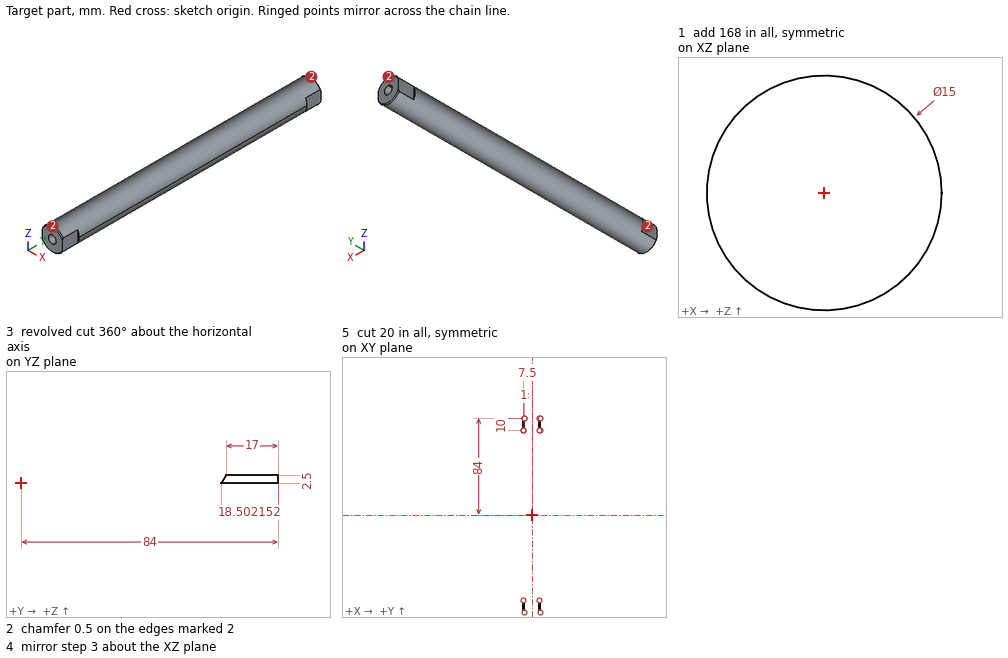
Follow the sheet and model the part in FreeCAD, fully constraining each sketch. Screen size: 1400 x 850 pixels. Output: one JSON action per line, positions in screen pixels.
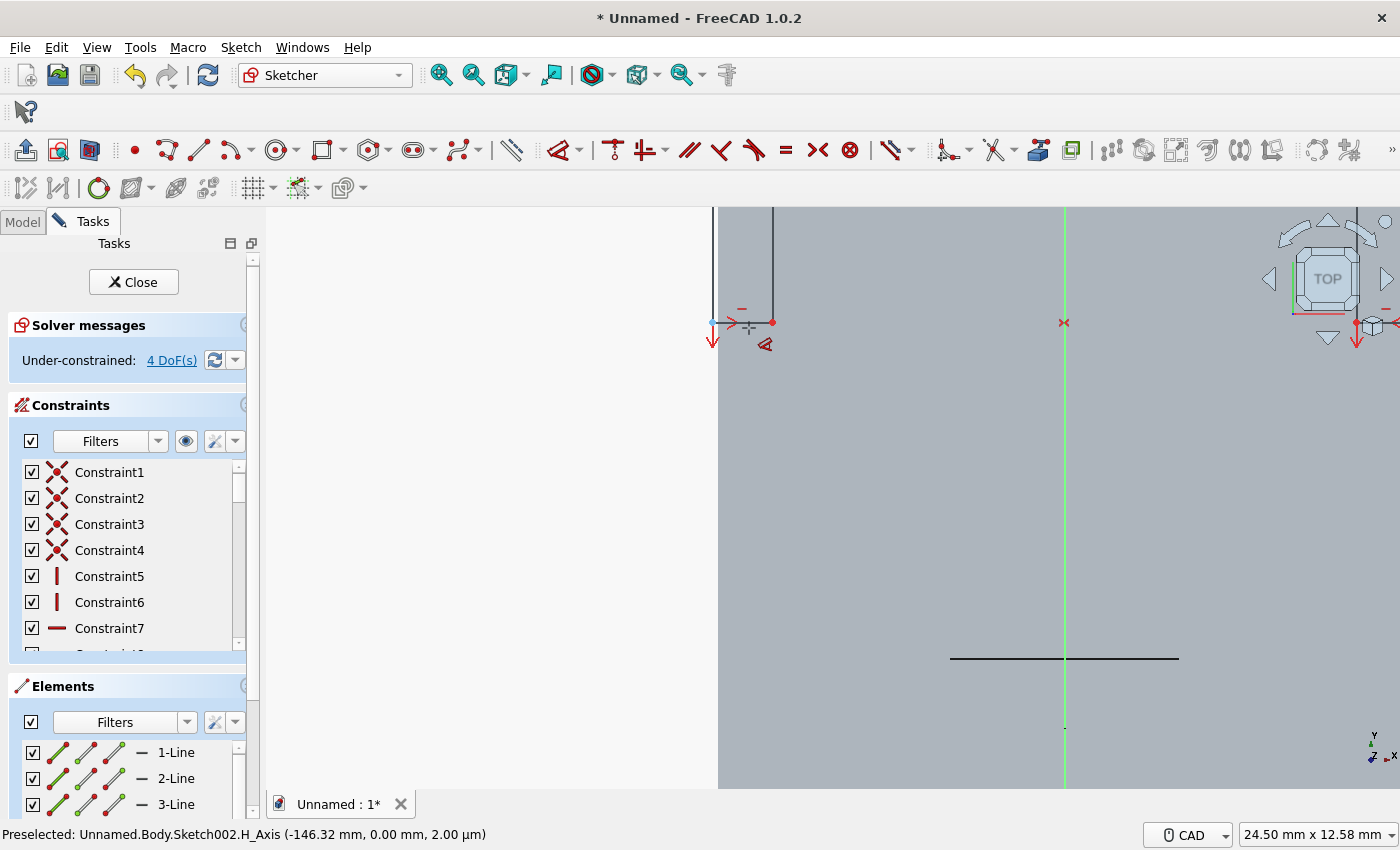
{"action": "left_click", "coordinate": [743, 323]}
{"action": "left_click", "coordinate": [743, 289]}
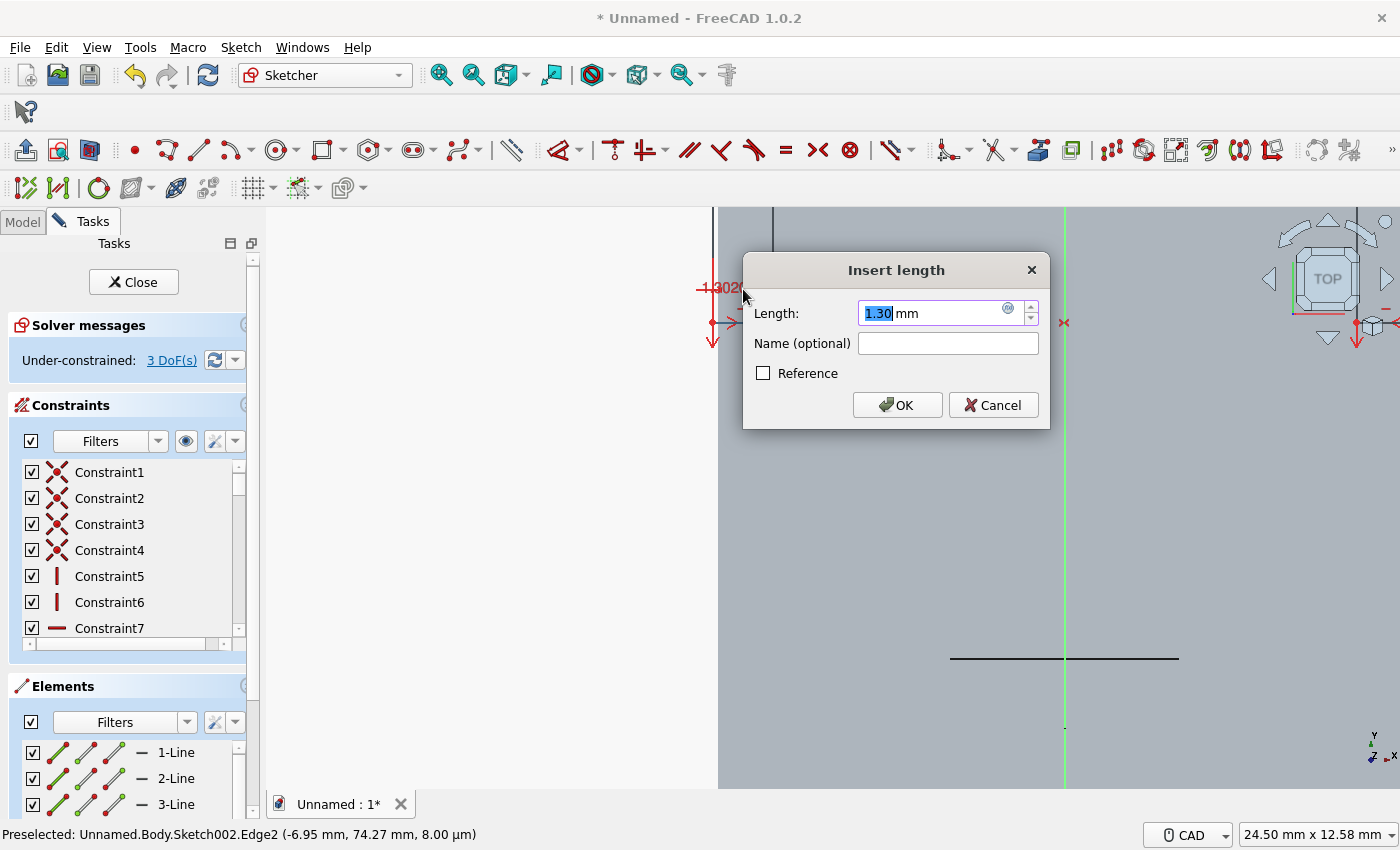
{"action": "type", "text": "1"}
{"action": "key", "text": "Return"}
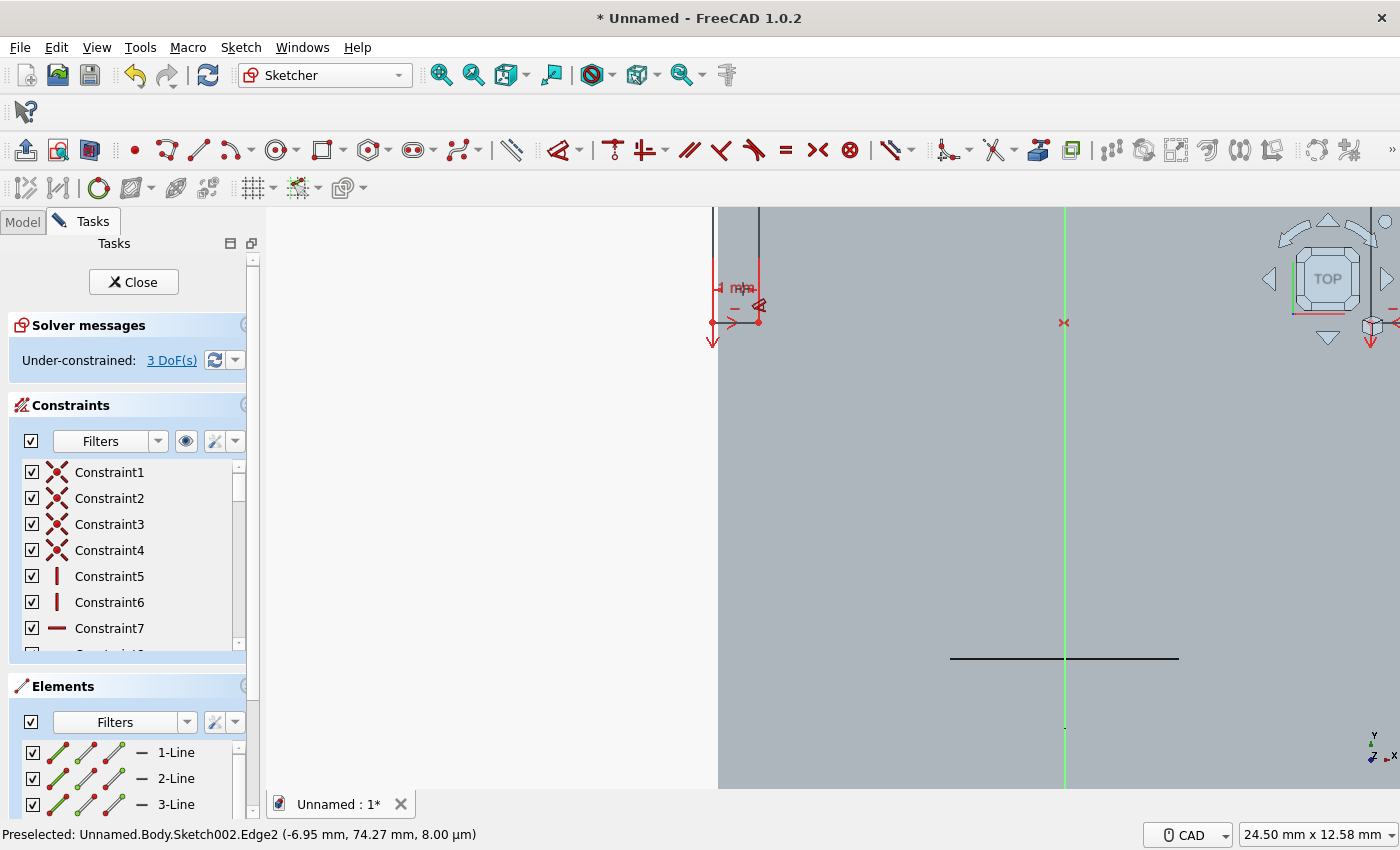
{"action": "scroll", "coordinate": [749, 327], "scroll_direction": "down", "scroll_amount": 15}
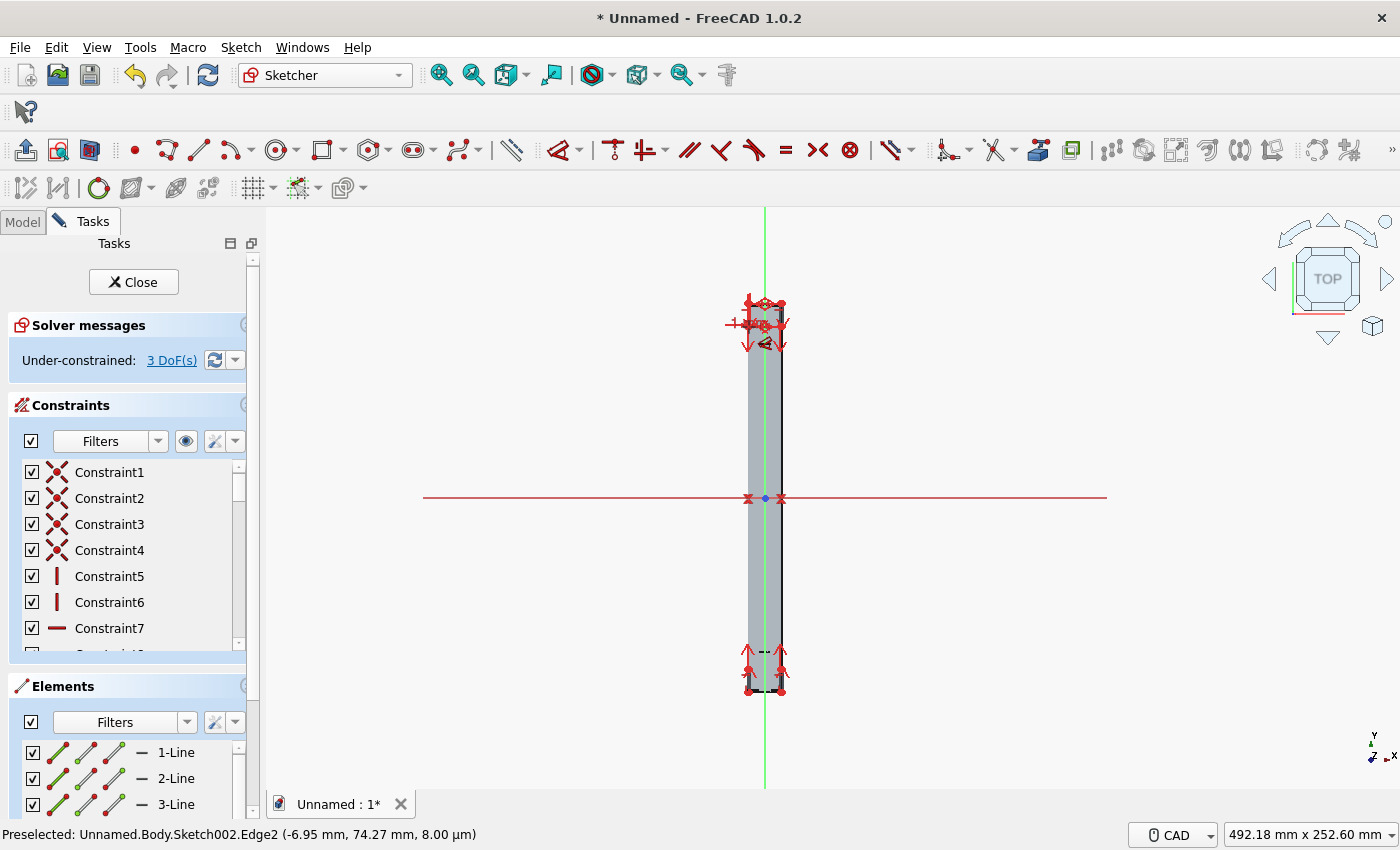
{"action": "scroll", "coordinate": [748, 311], "scroll_direction": "up", "scroll_amount": 9}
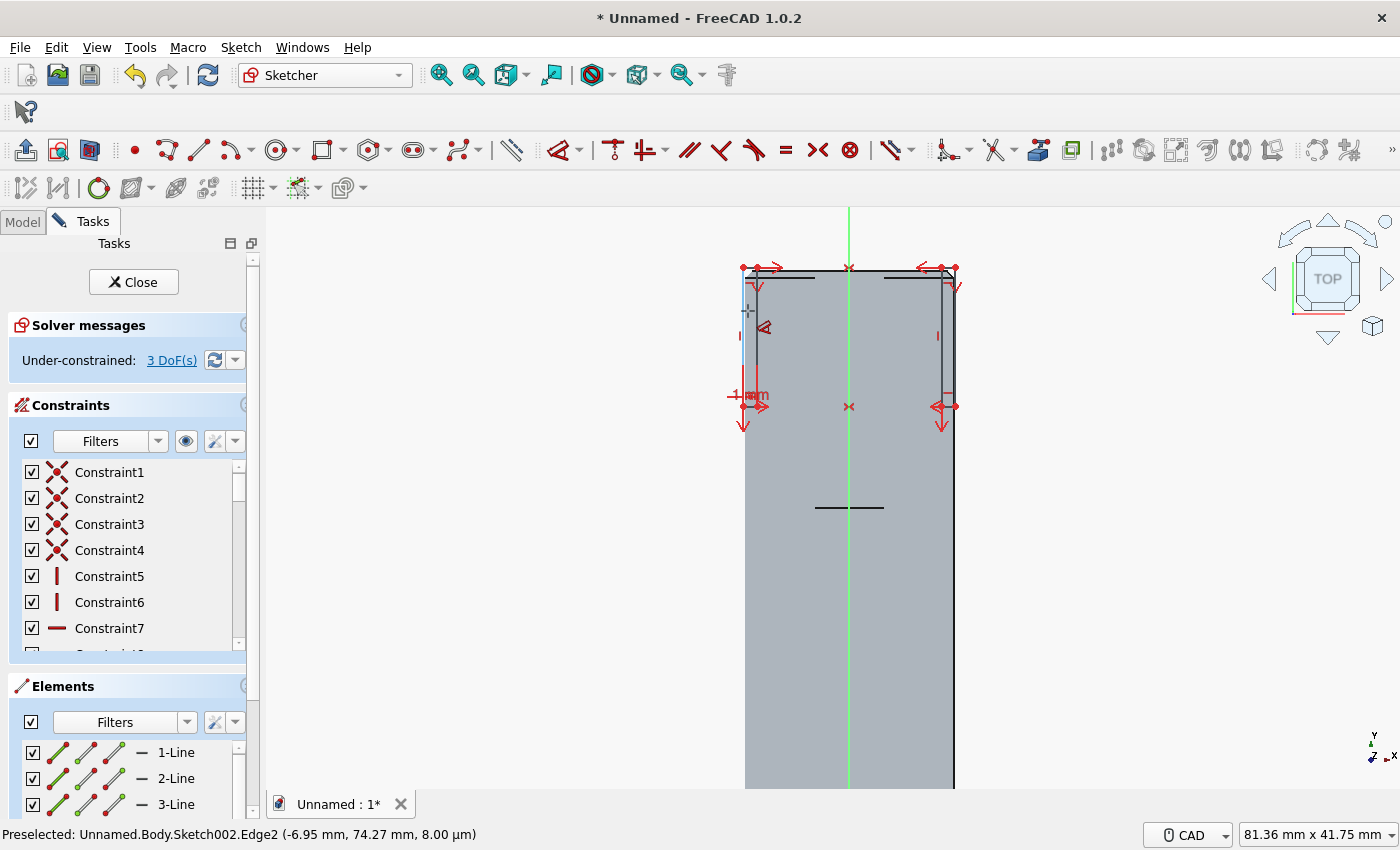
{"action": "left_click", "coordinate": [743, 309]}
{"action": "left_click", "coordinate": [709, 337]}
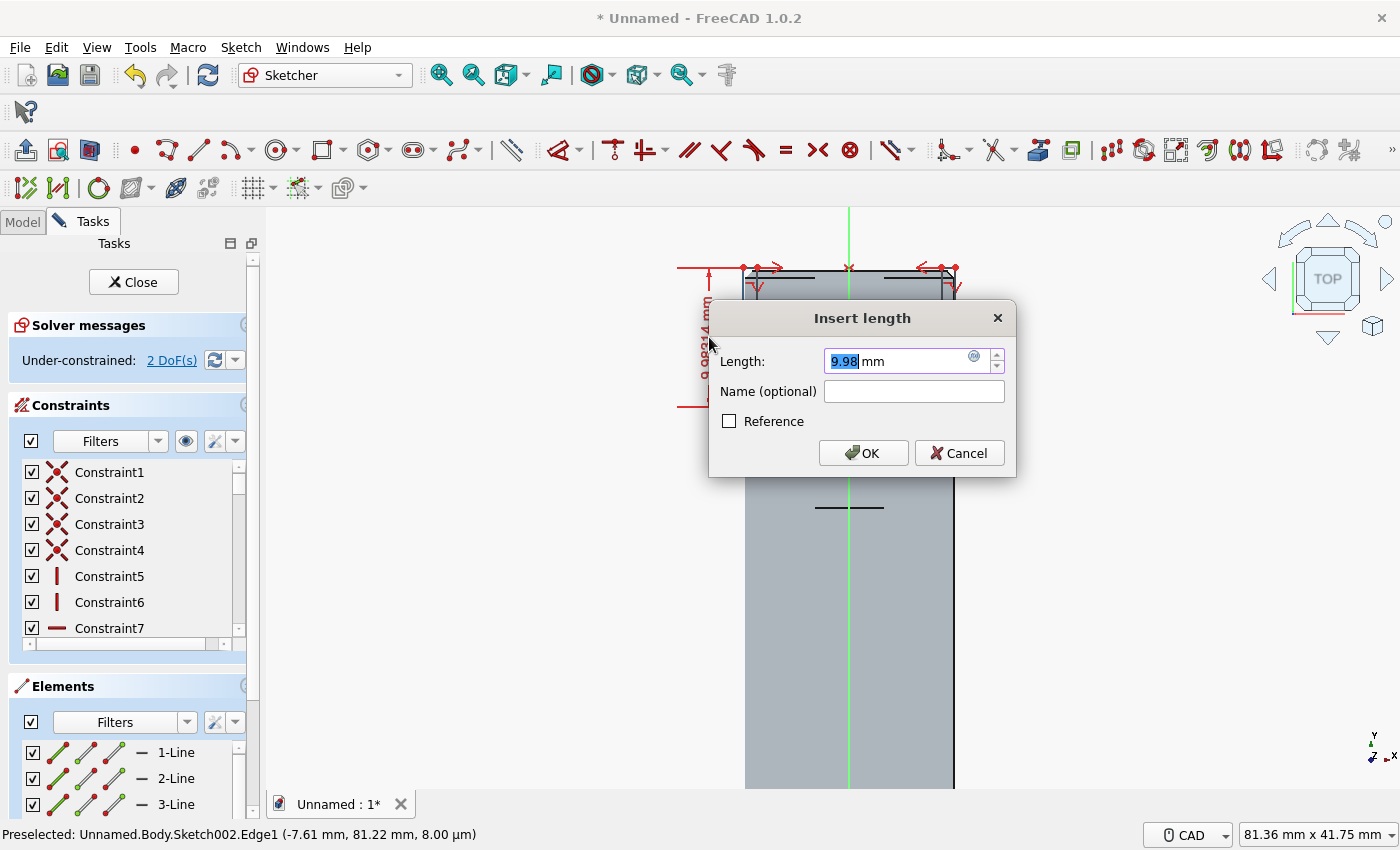
{"action": "type", "text": "10"}
{"action": "key", "text": "Return"}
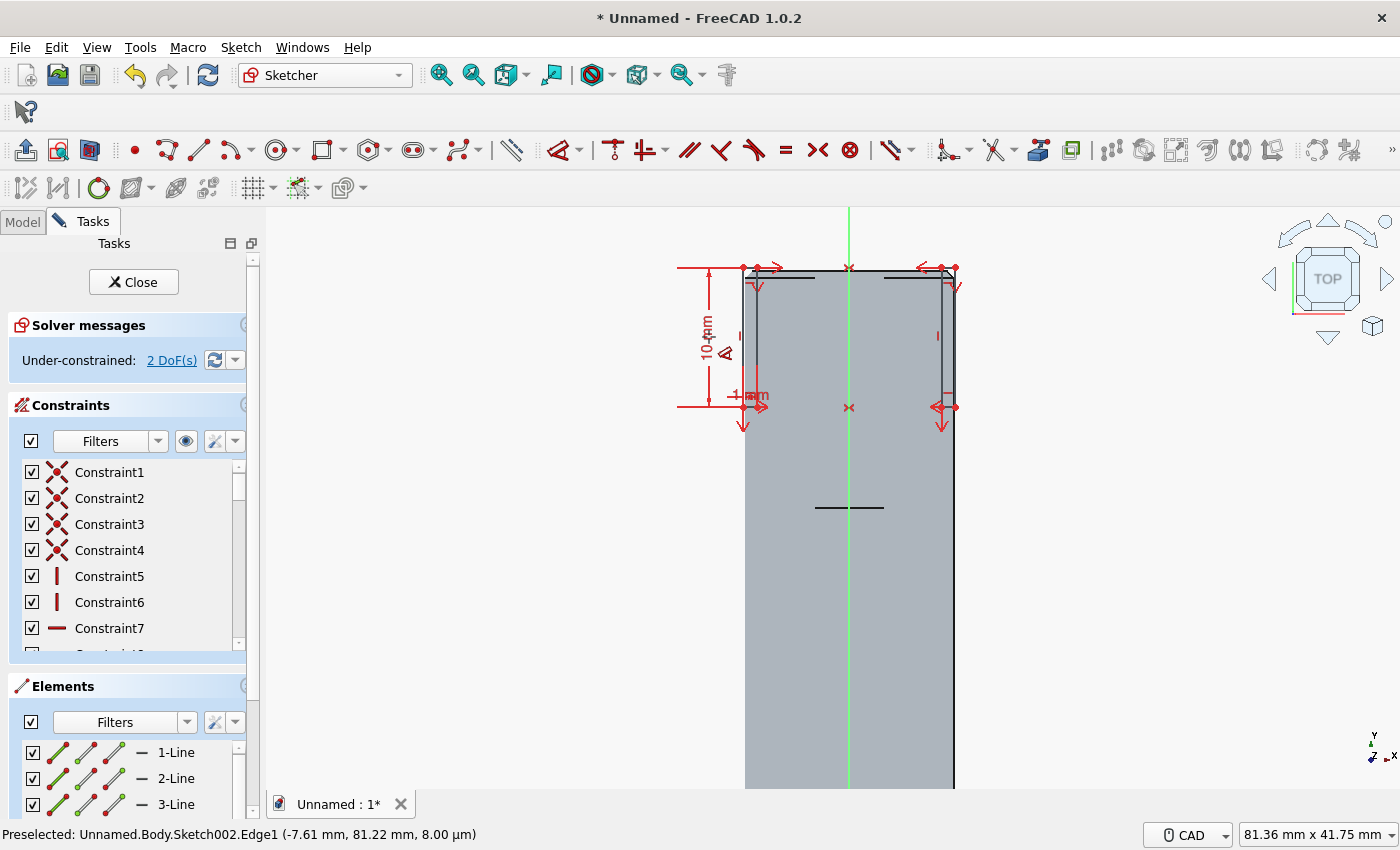
{"action": "left_click", "coordinate": [743, 268]}
{"action": "left_click", "coordinate": [709, 514]}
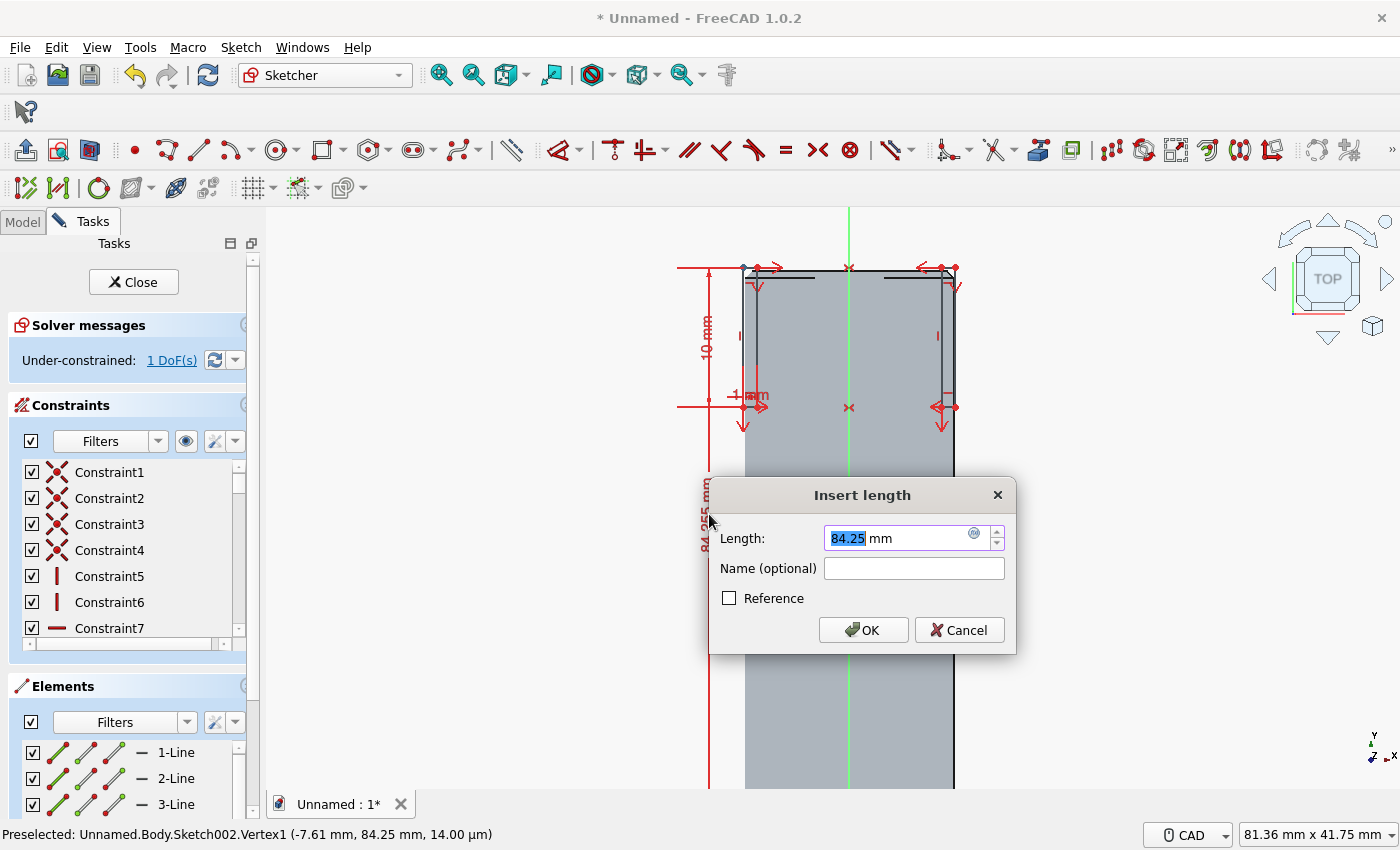
{"action": "type", "text": "84"}
{"action": "key", "text": "Return"}